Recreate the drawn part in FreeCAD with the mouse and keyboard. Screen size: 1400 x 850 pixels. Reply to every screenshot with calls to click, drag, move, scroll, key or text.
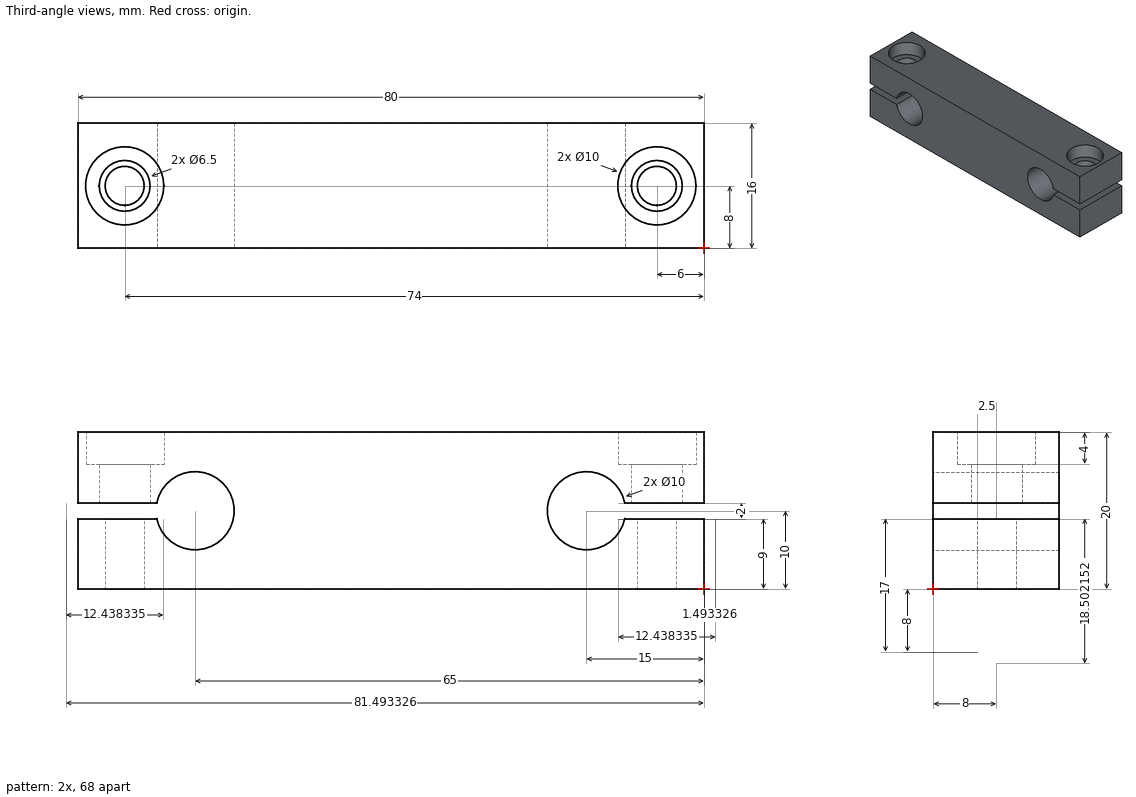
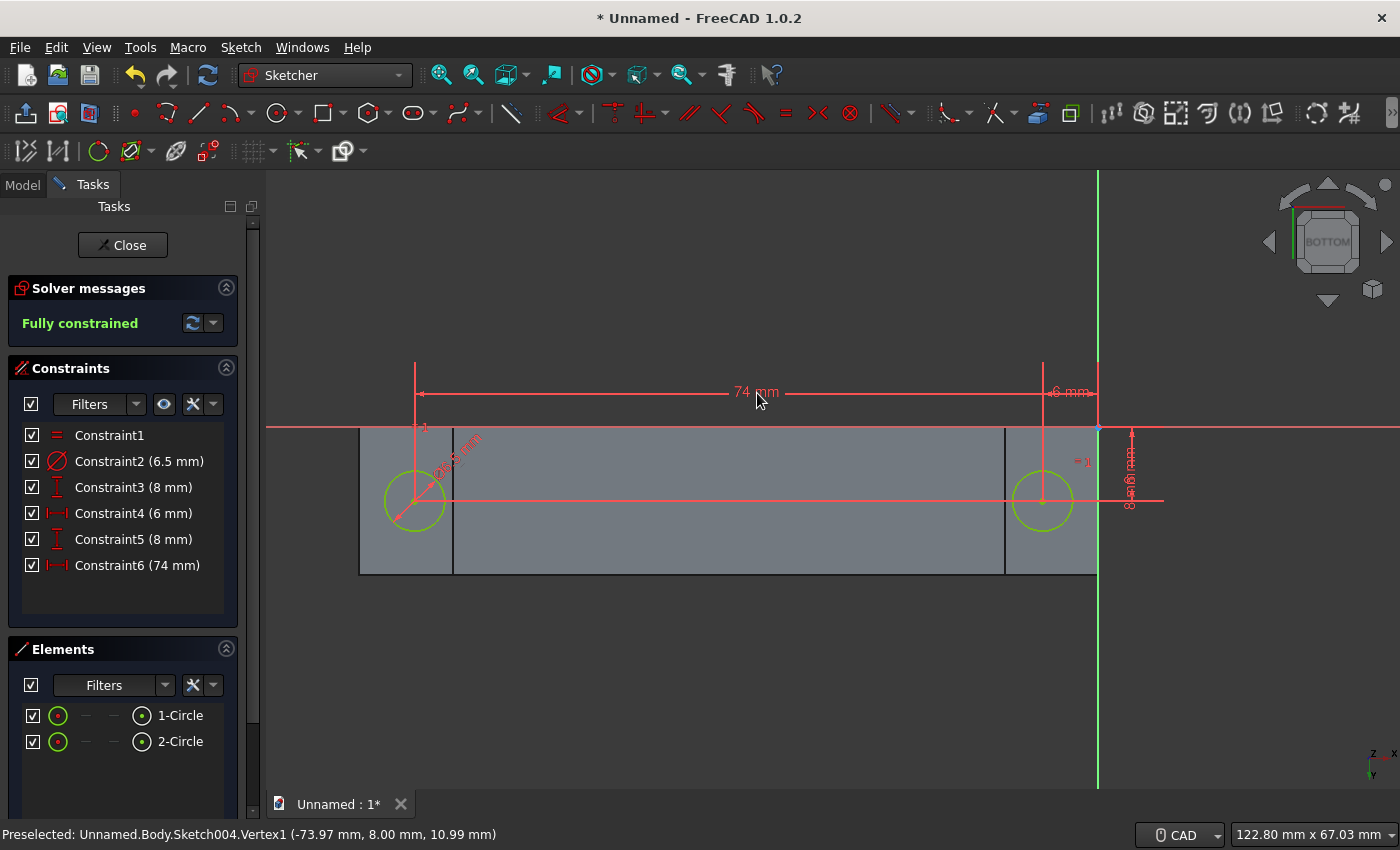
click(123, 245)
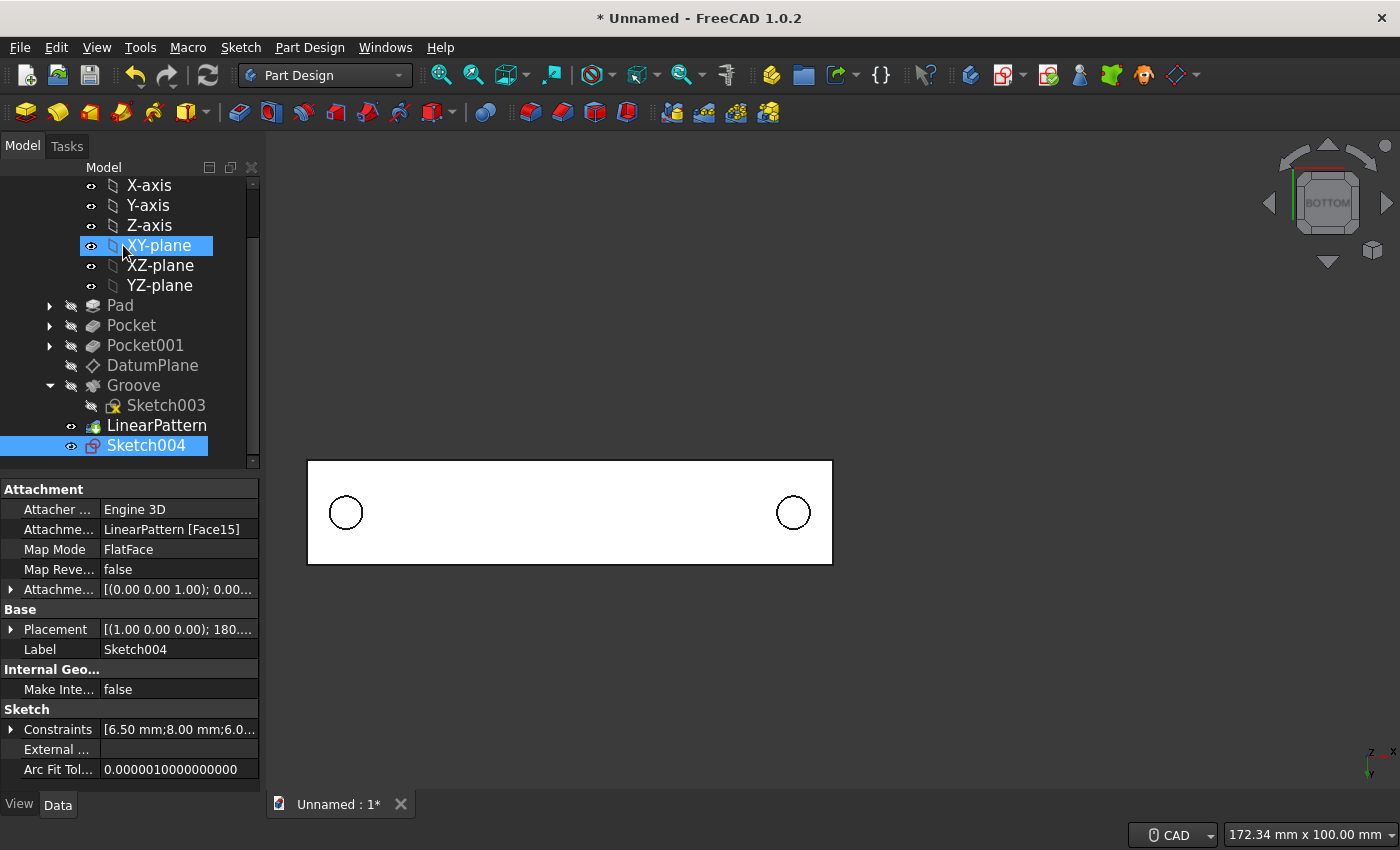
click(240, 112)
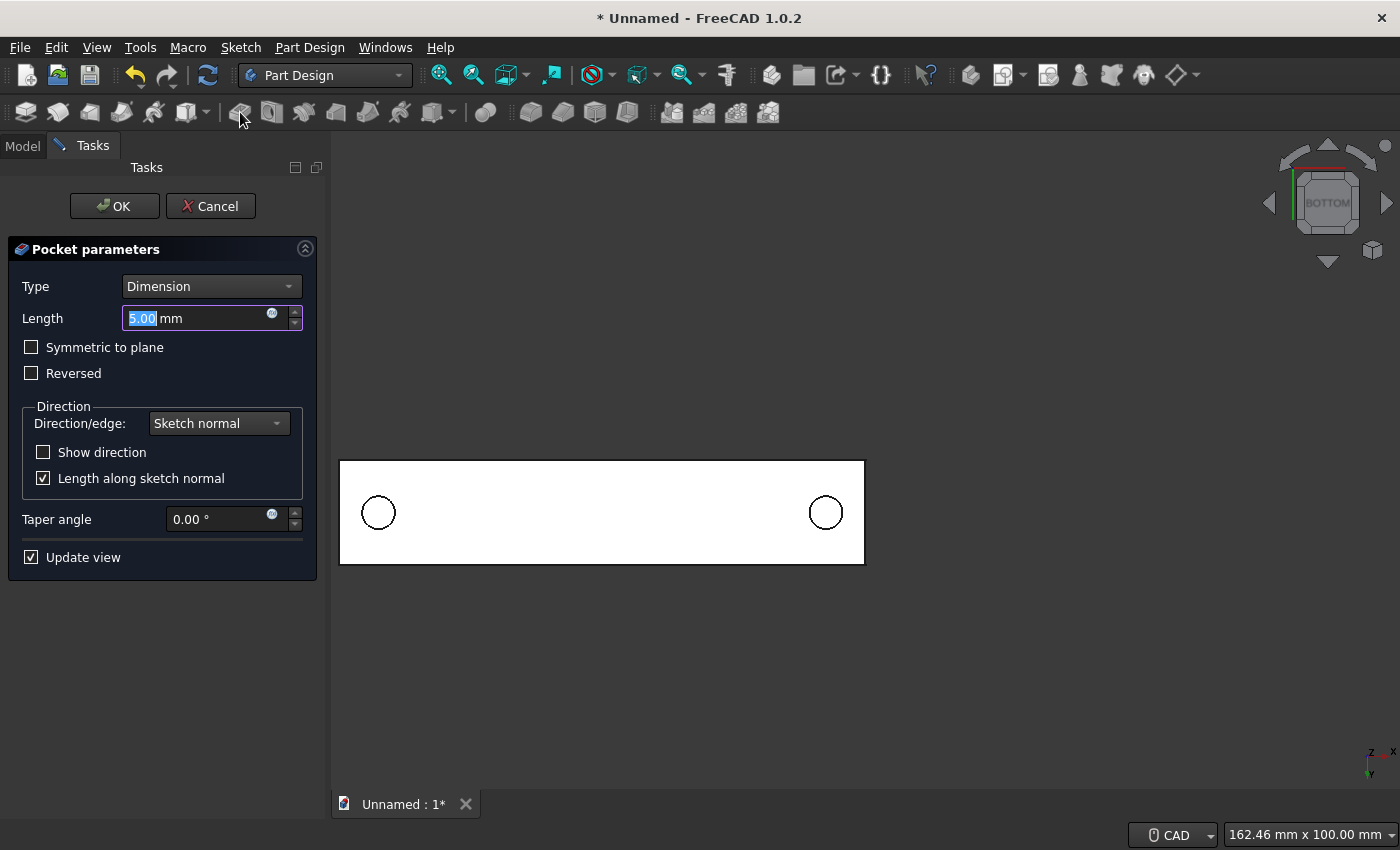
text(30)
key(Tab)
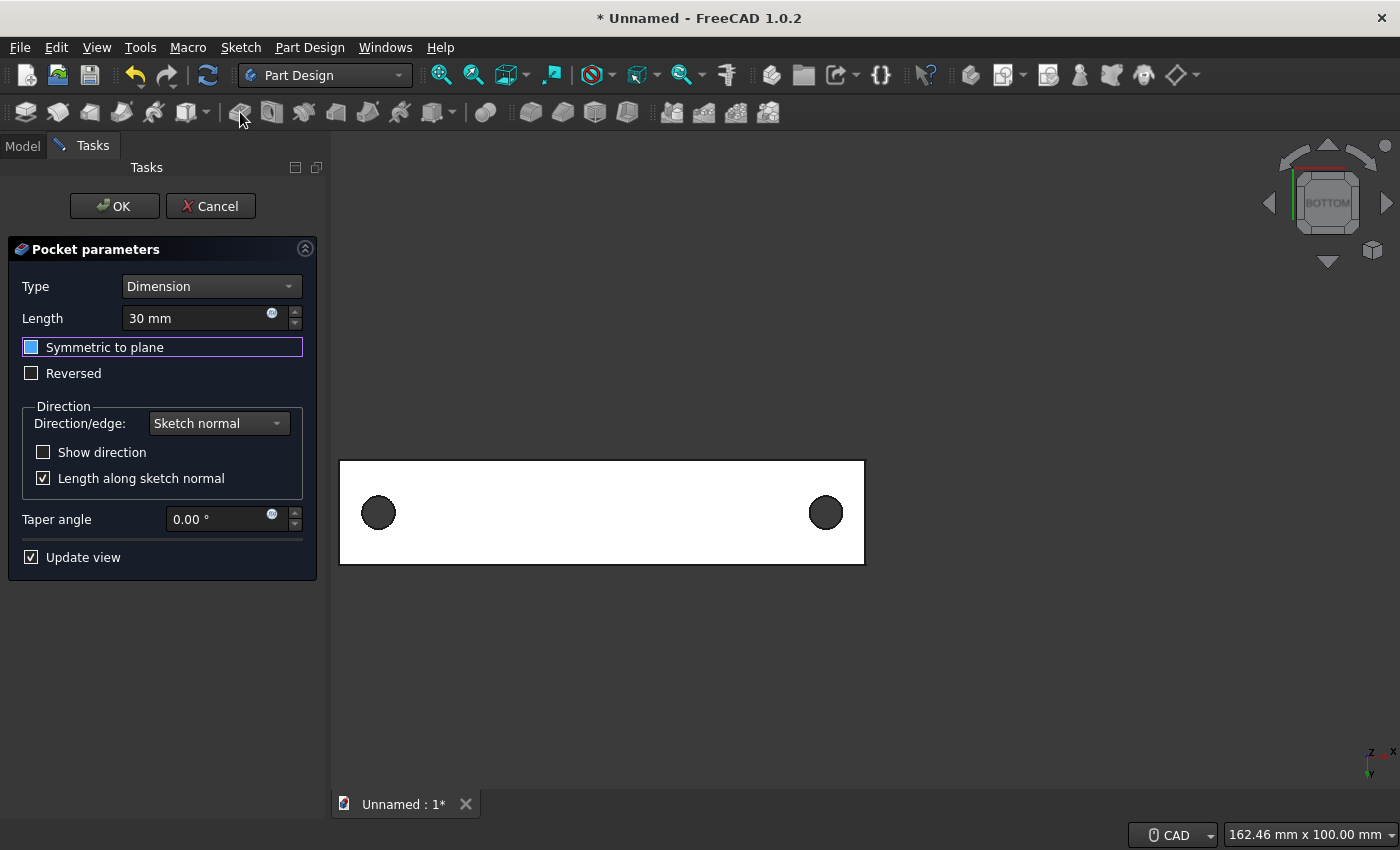
click(115, 206)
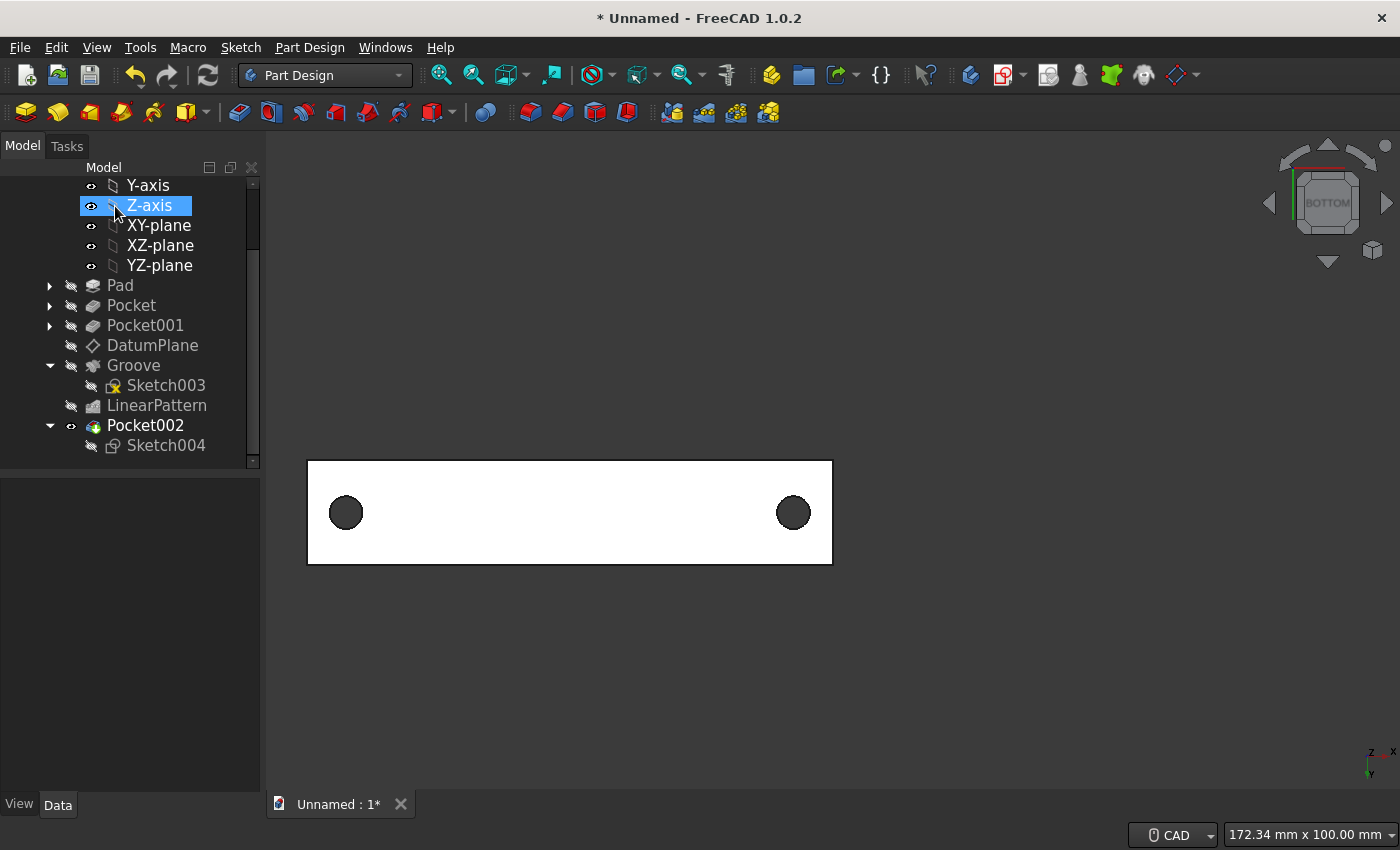
key(0)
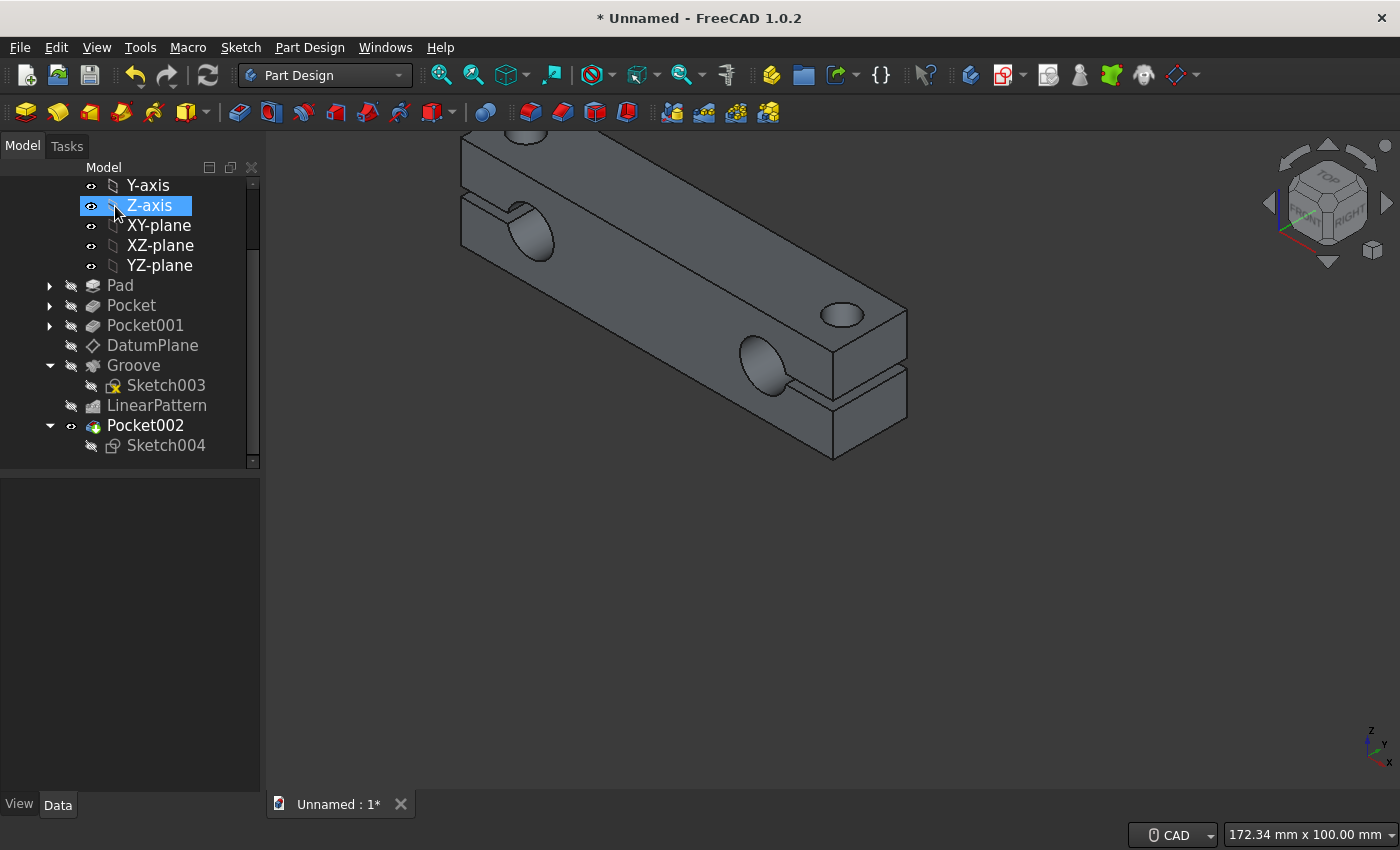
click(442, 76)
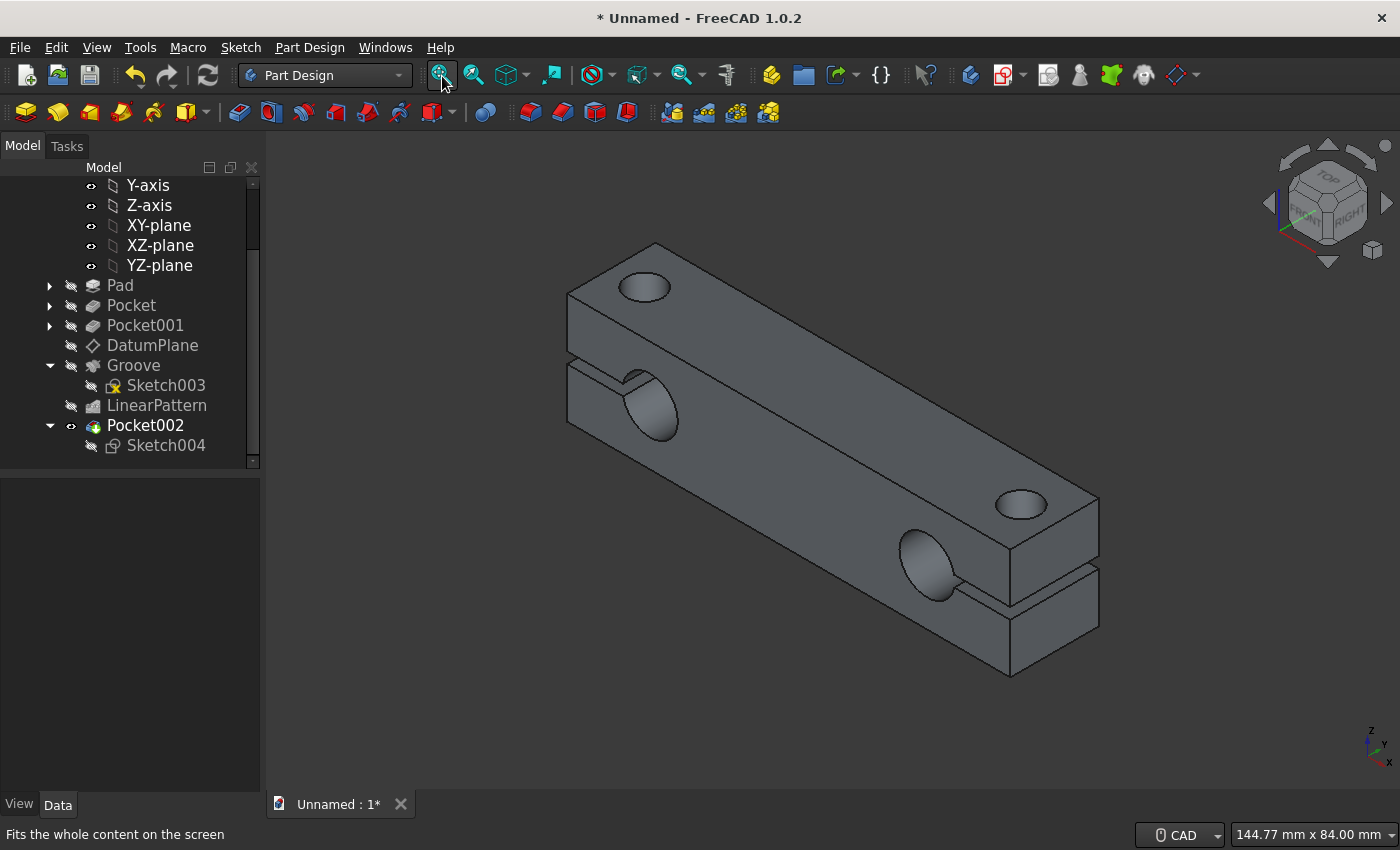
click(896, 432)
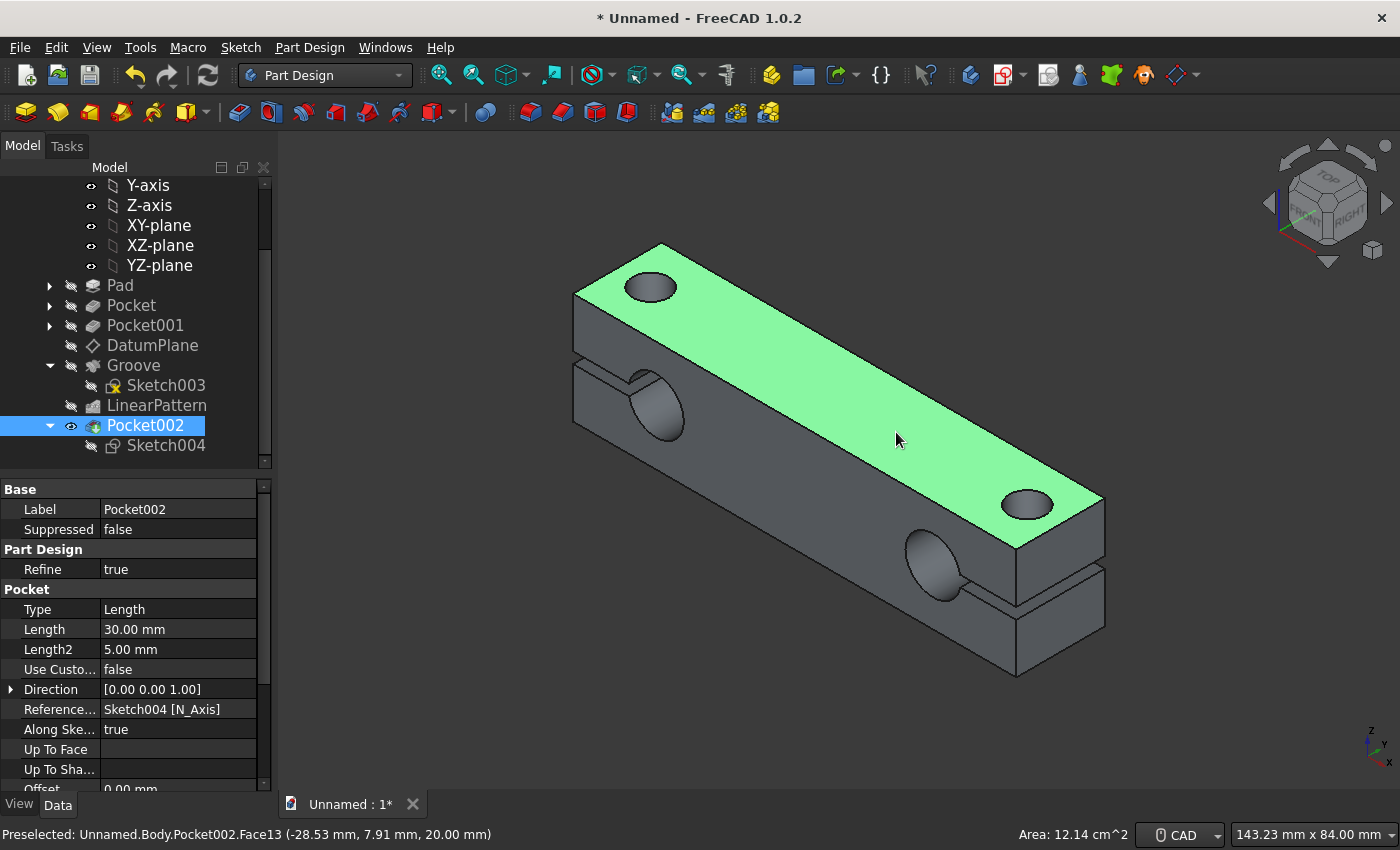
click(1004, 76)